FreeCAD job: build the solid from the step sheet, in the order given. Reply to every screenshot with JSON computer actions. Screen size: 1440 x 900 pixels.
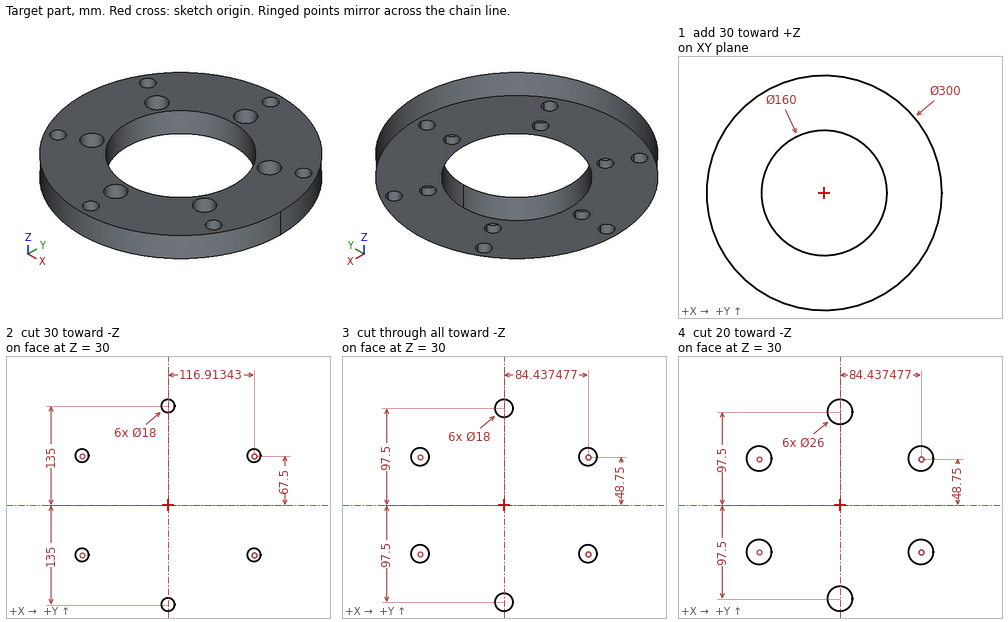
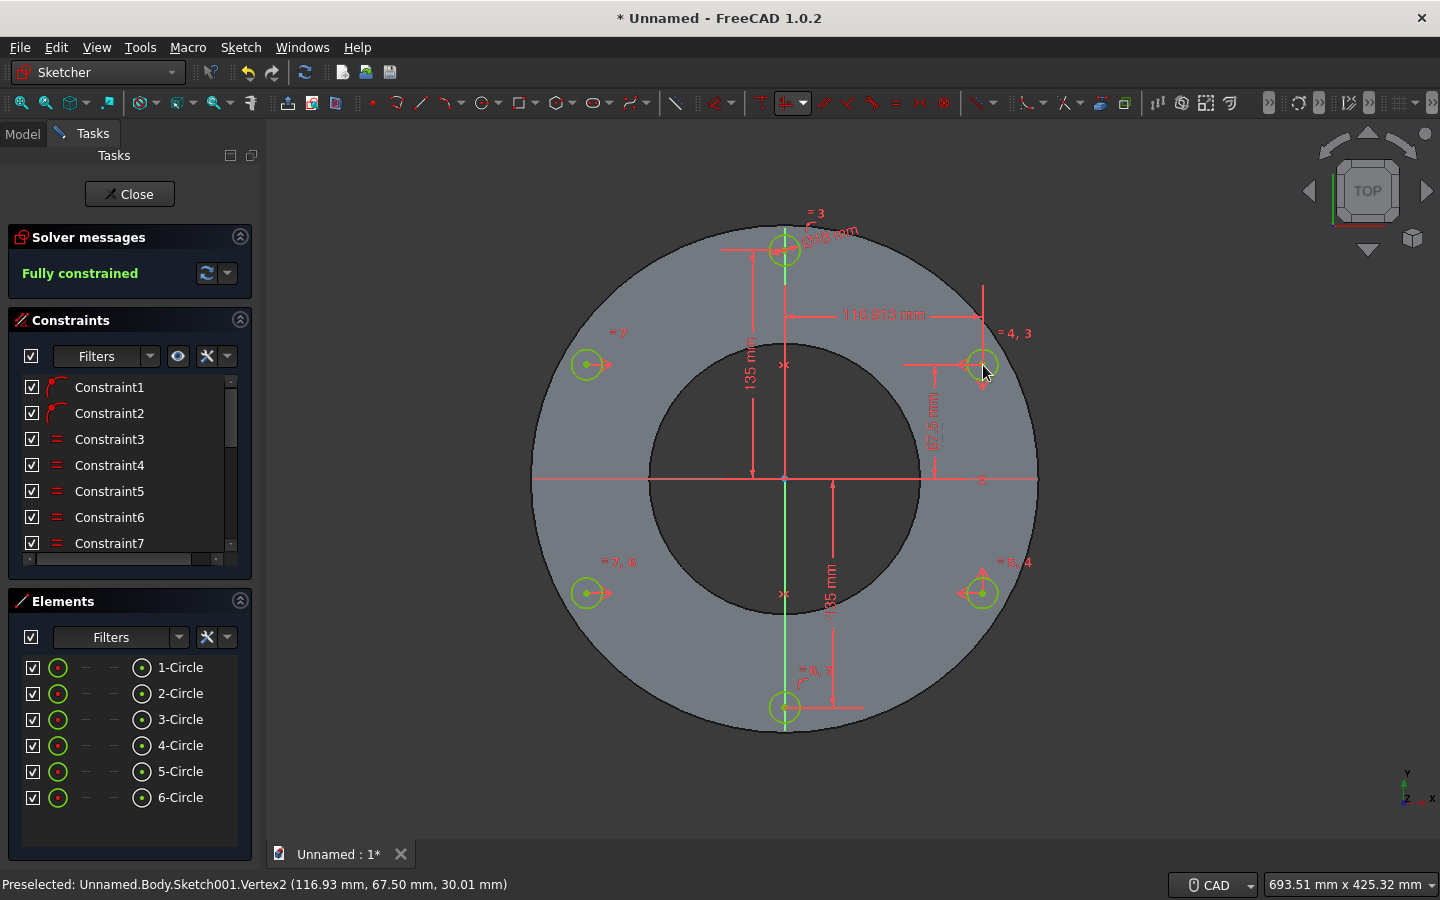
{"action": "left_click", "coordinate": [130, 194]}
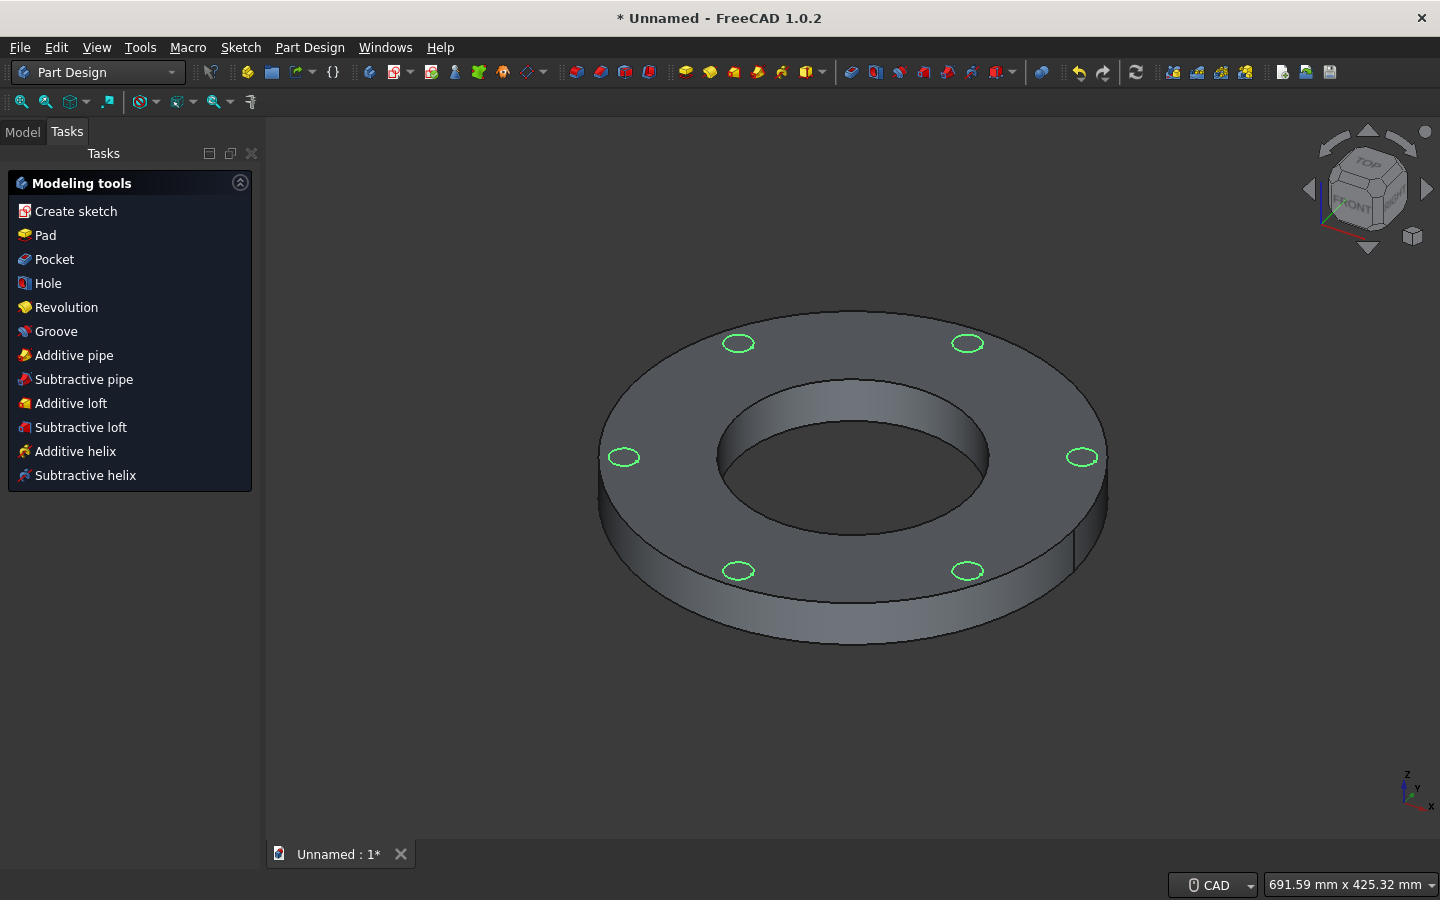
{"action": "left_click", "coordinate": [852, 72]}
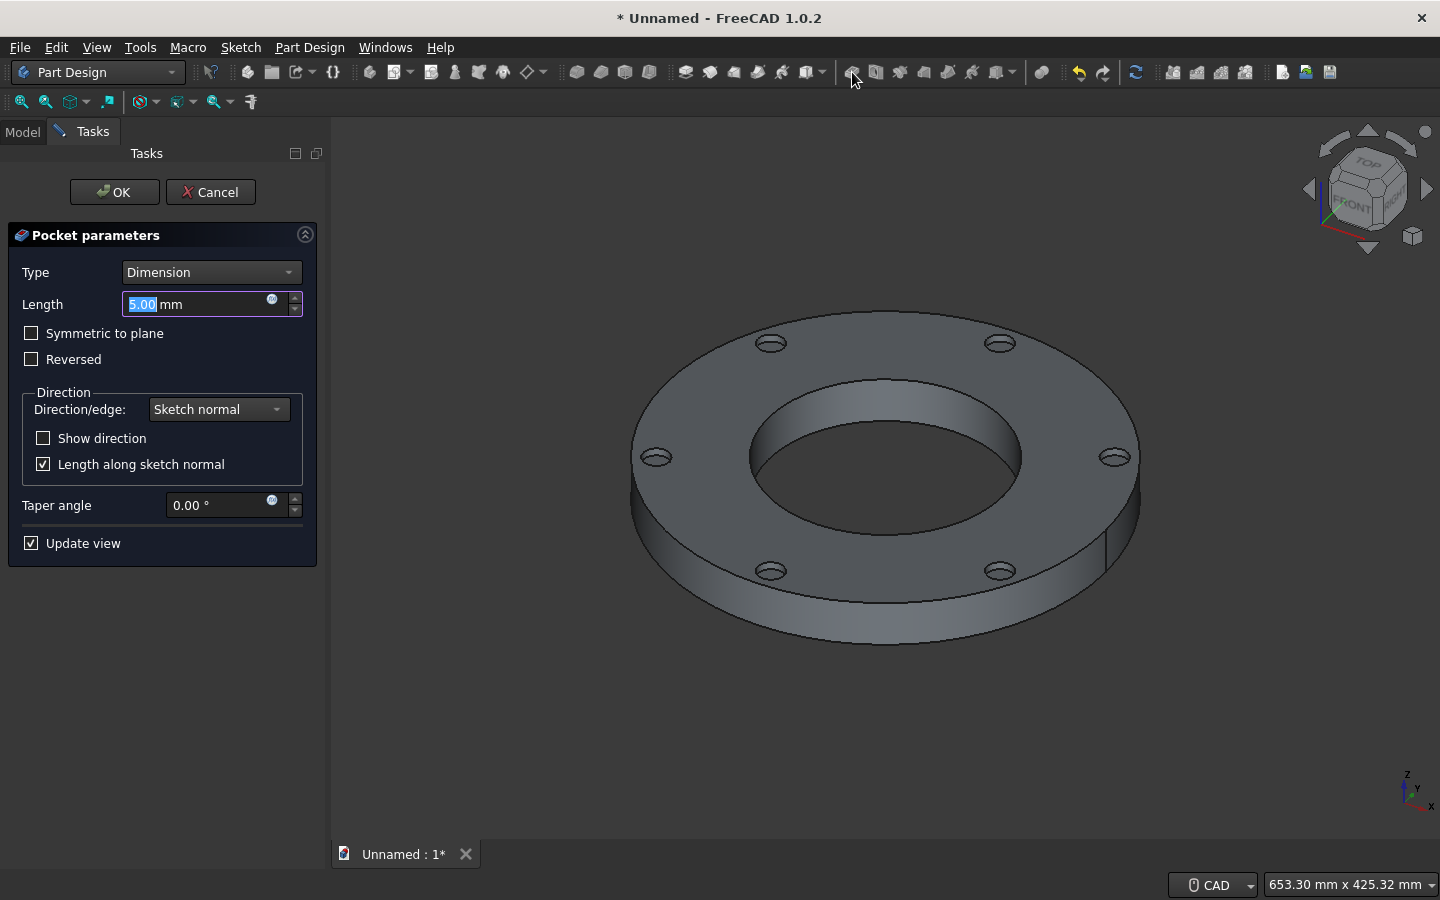
{"action": "type", "text": "30"}
{"action": "key", "text": "Tab"}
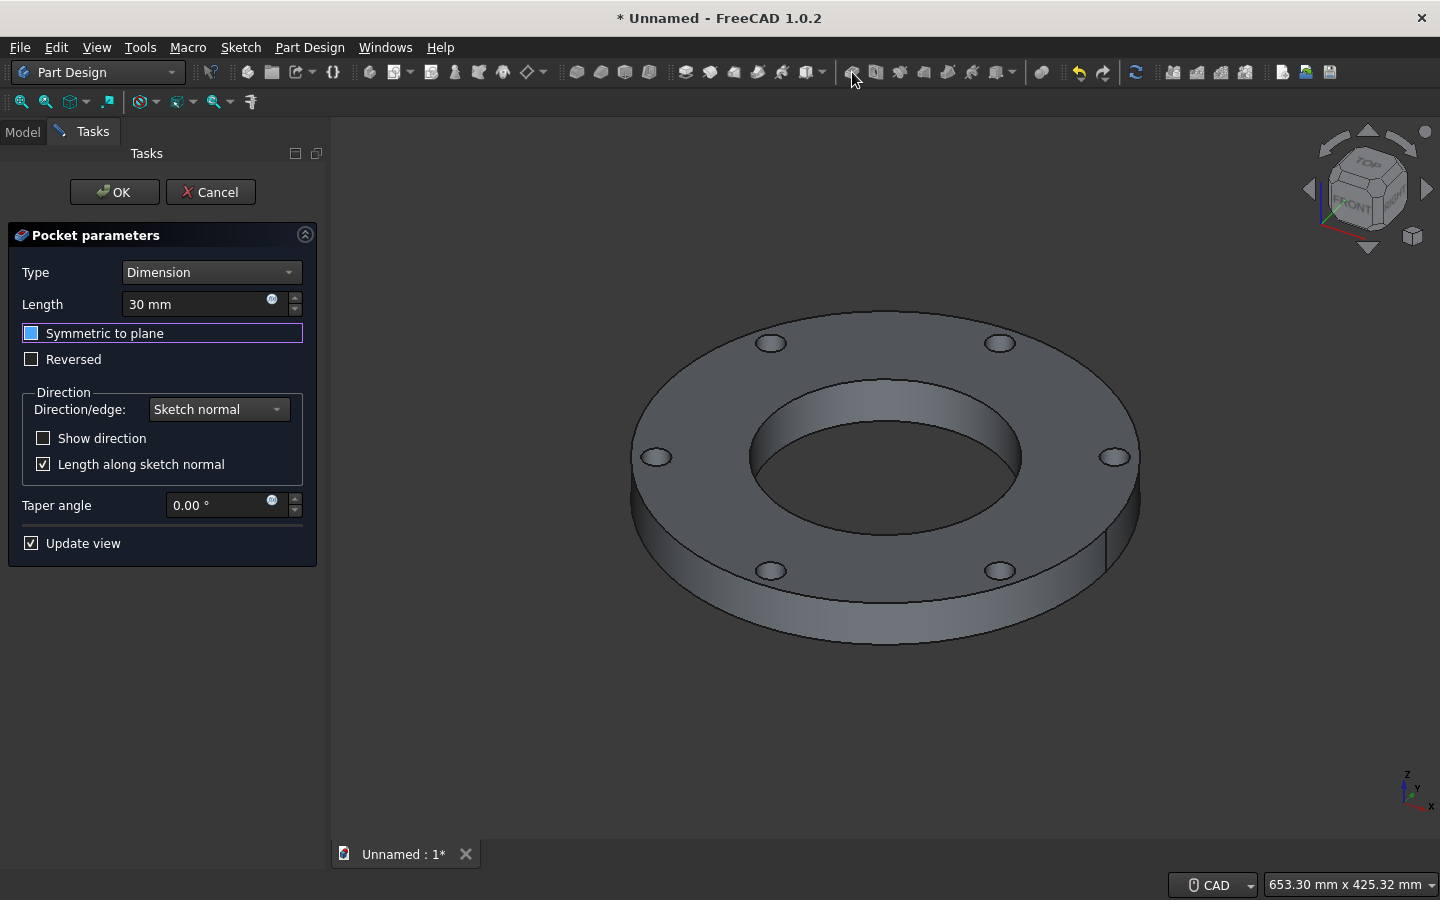
{"action": "left_click", "coordinate": [115, 192]}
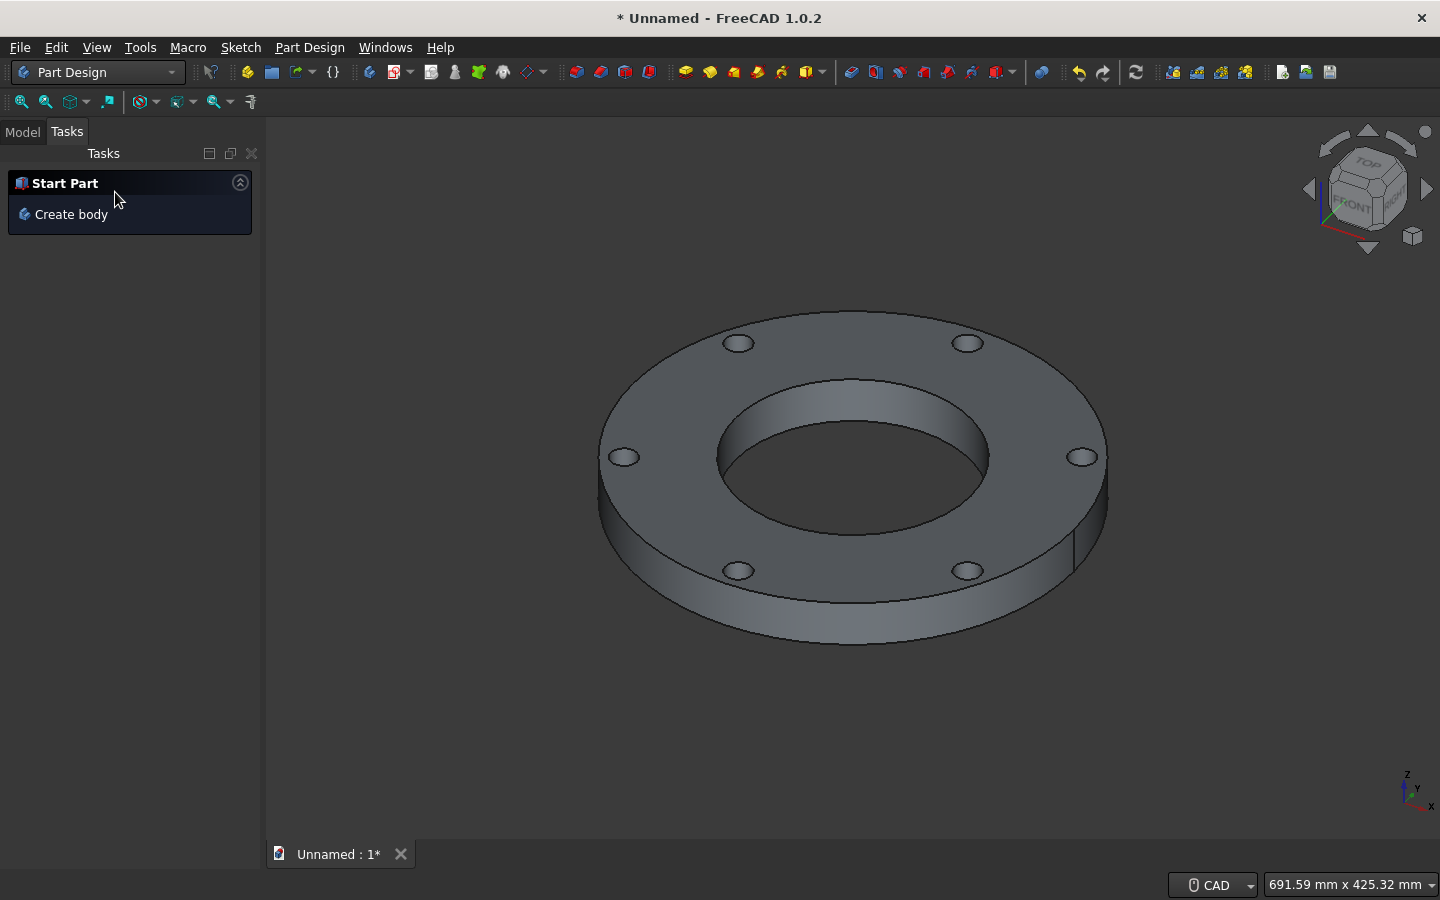
{"action": "left_click", "coordinate": [1052, 426]}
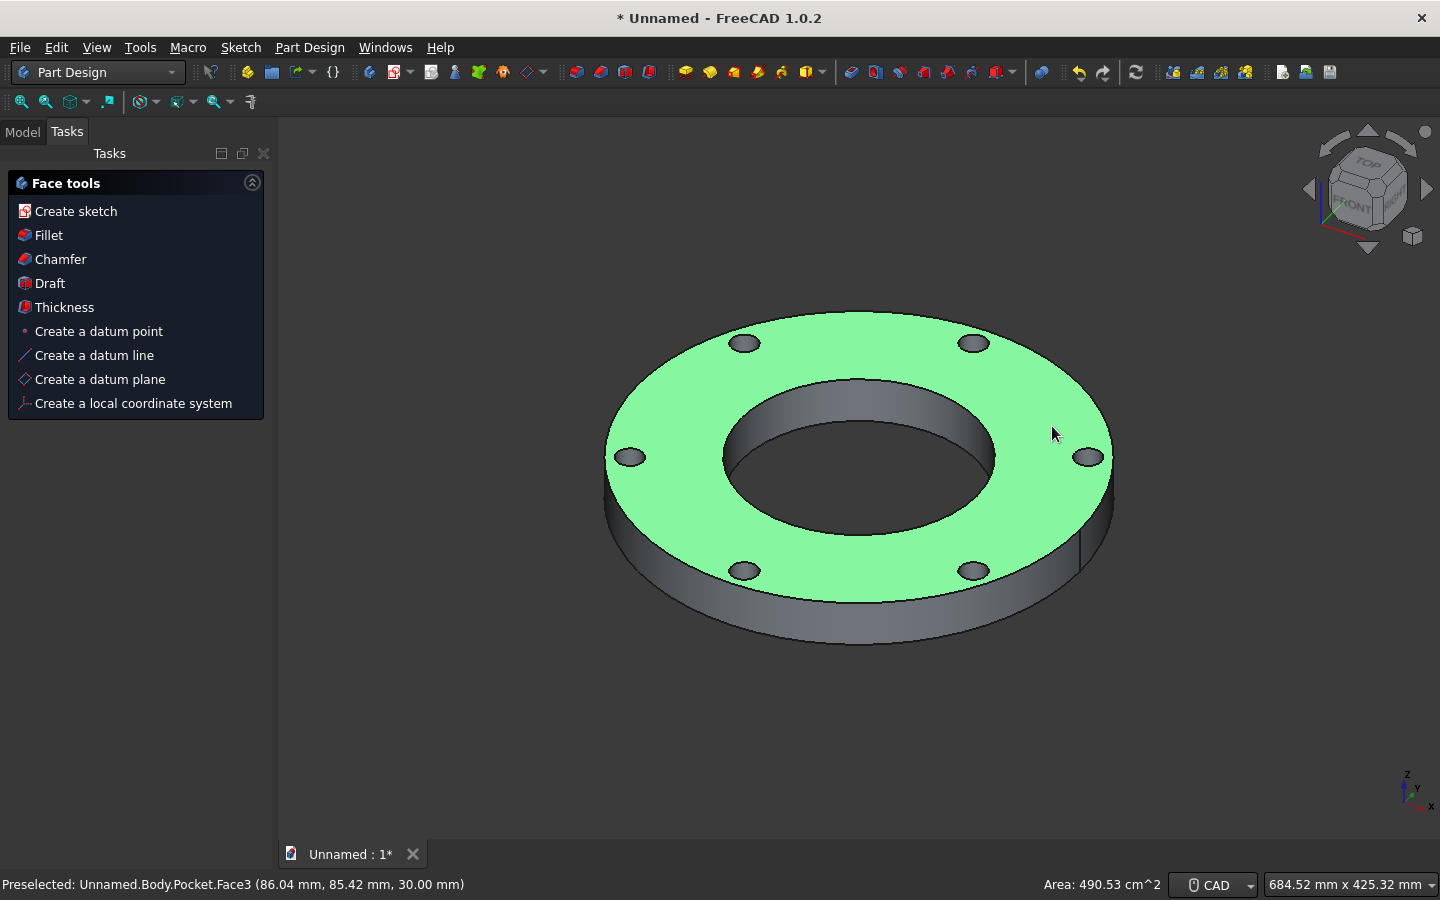
{"action": "left_click", "coordinate": [394, 72]}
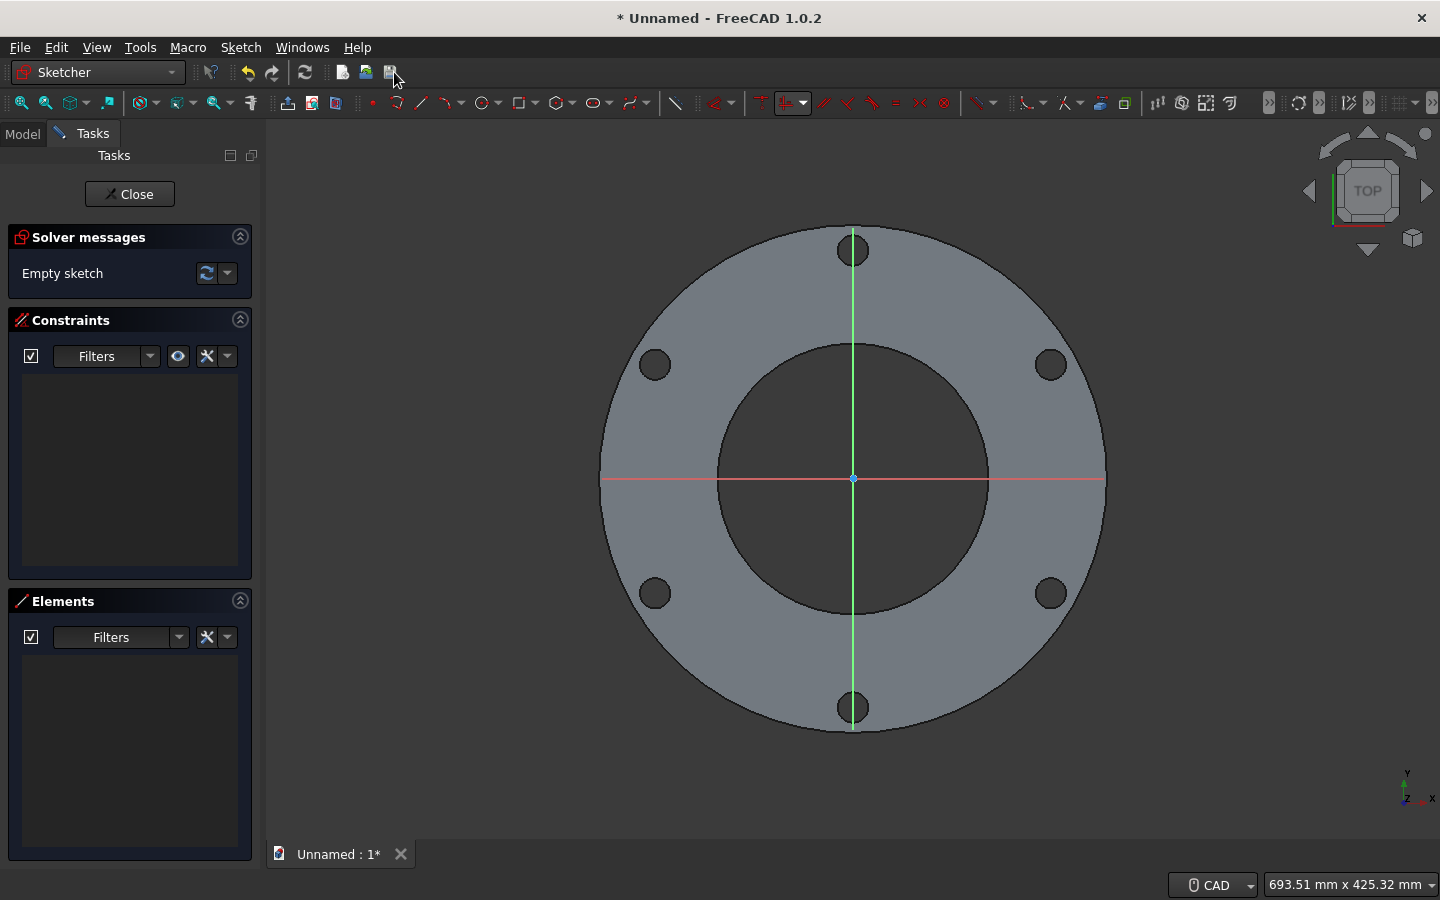
{"action": "key", "text": "g c"}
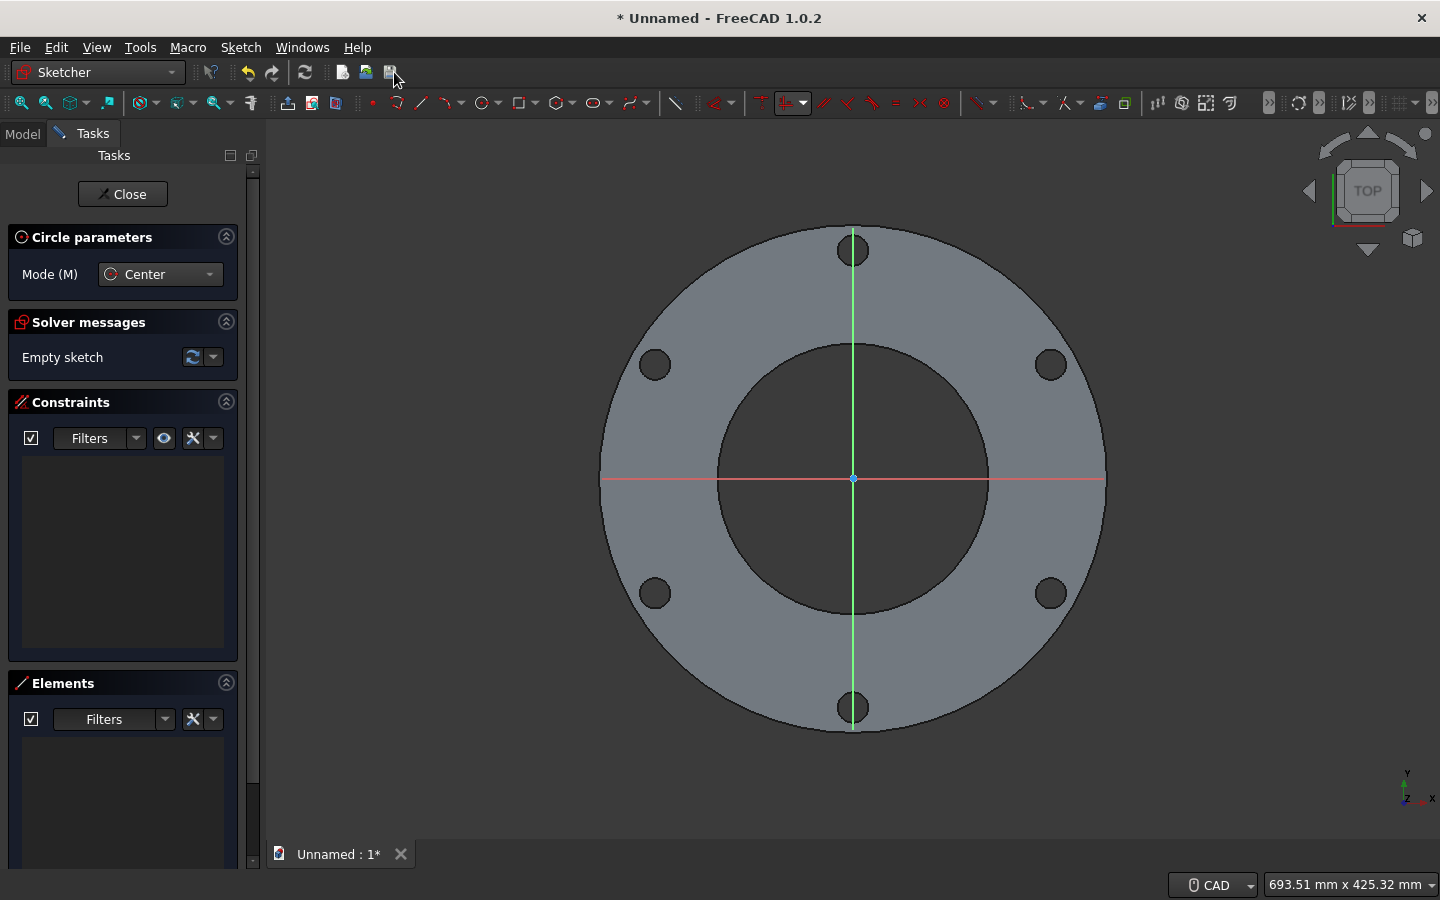
{"action": "scroll", "coordinate": [853, 314], "scroll_direction": "up", "scroll_amount": 2}